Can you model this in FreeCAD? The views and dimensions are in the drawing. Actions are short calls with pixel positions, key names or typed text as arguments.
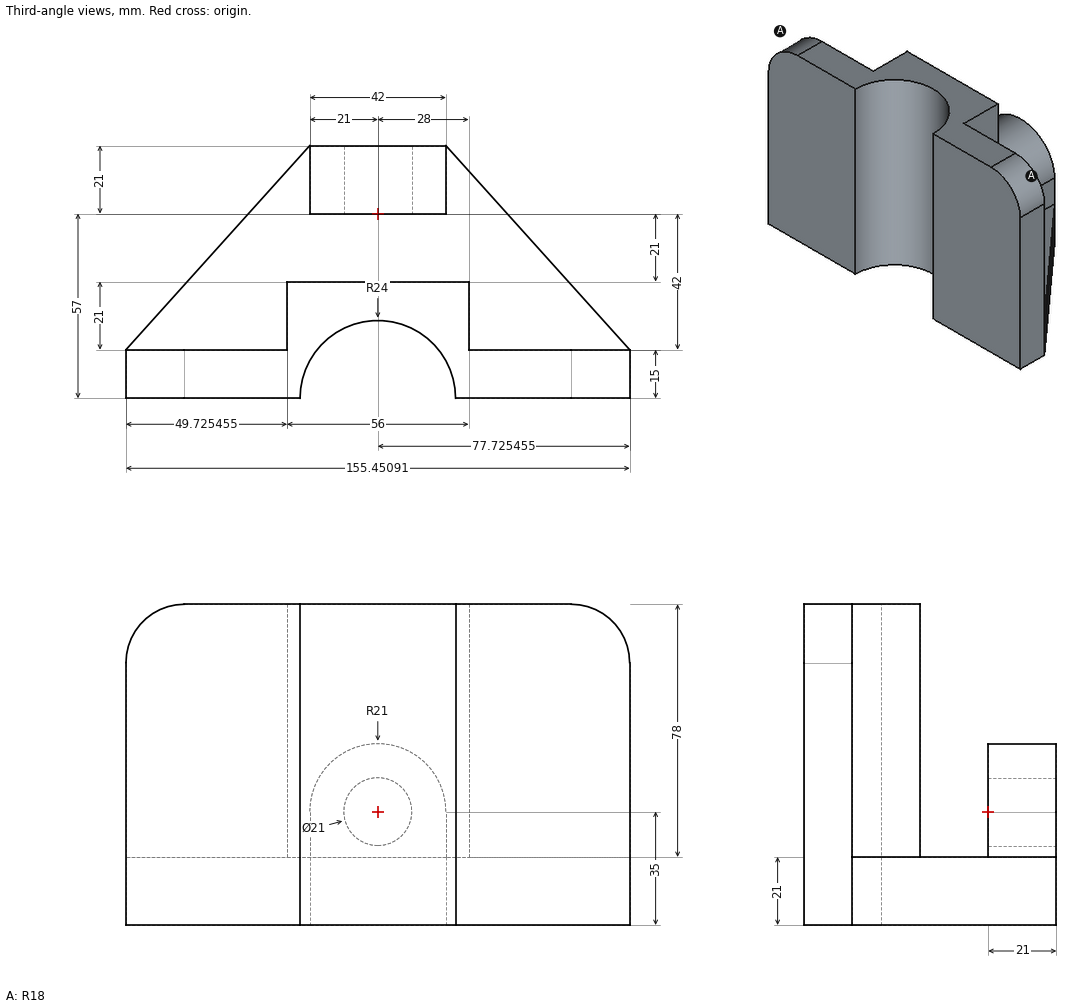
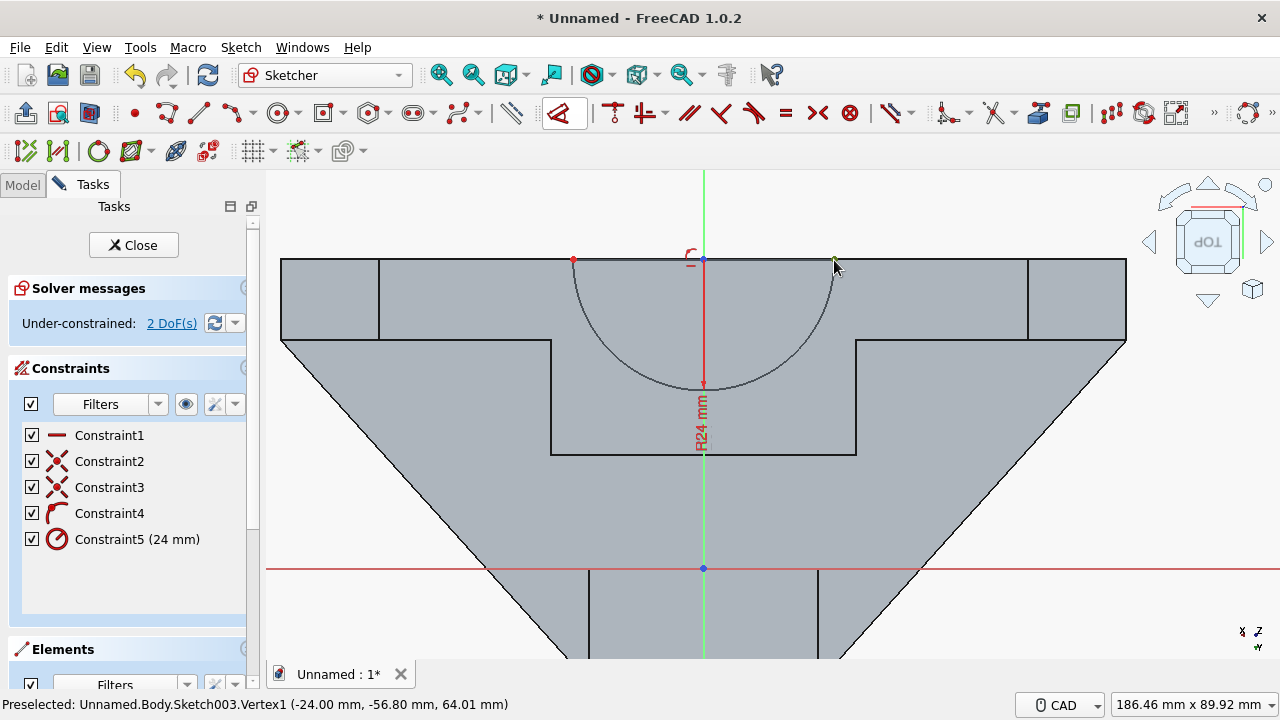
click(582, 114)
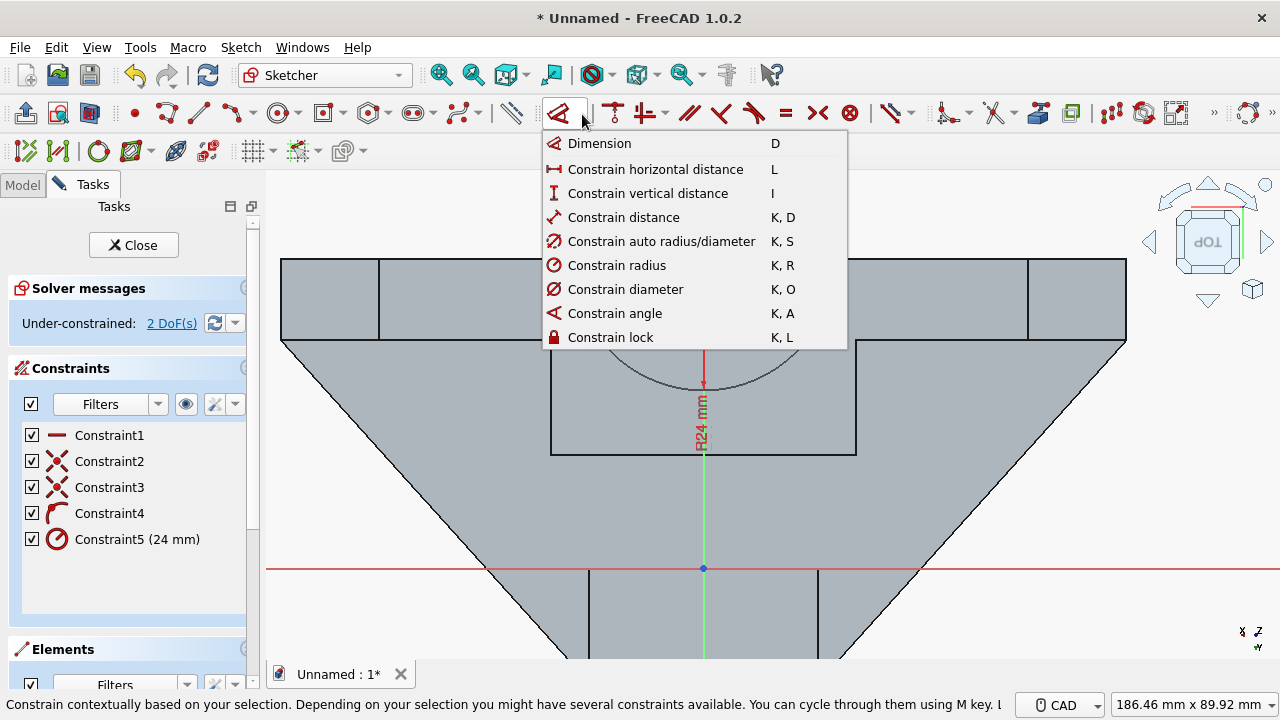
click(695, 193)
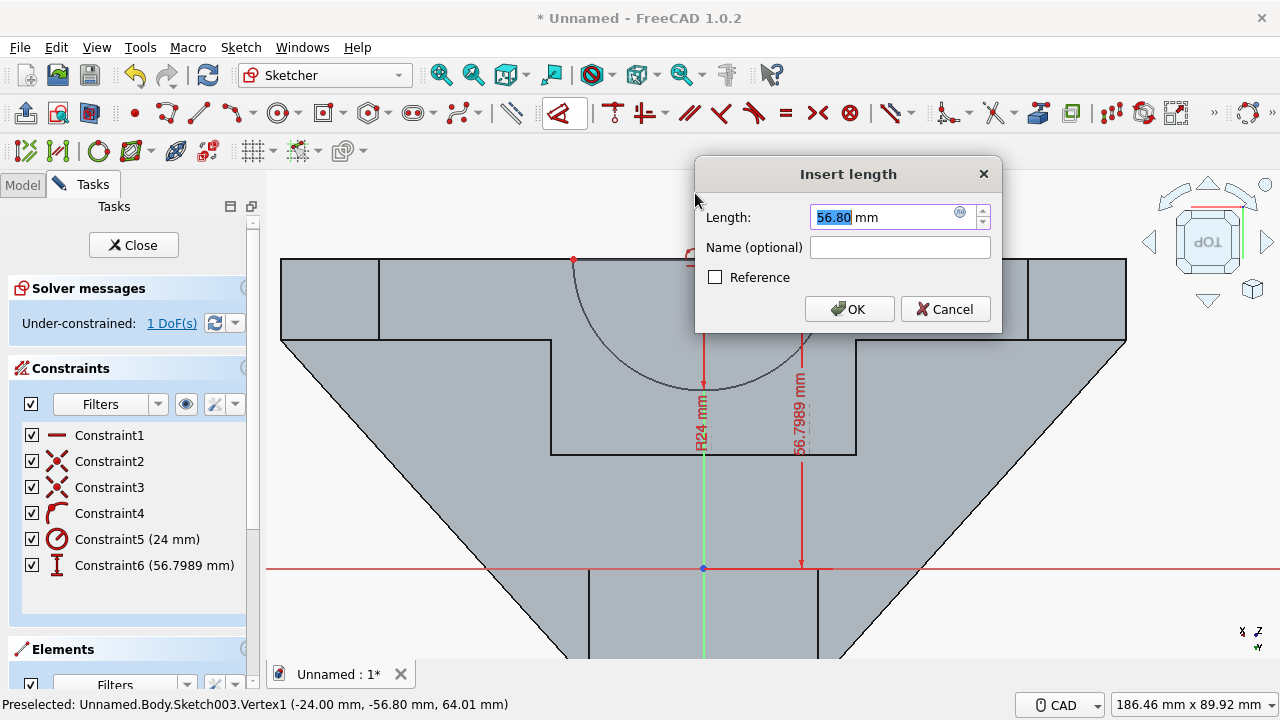
text(57)
key(Return)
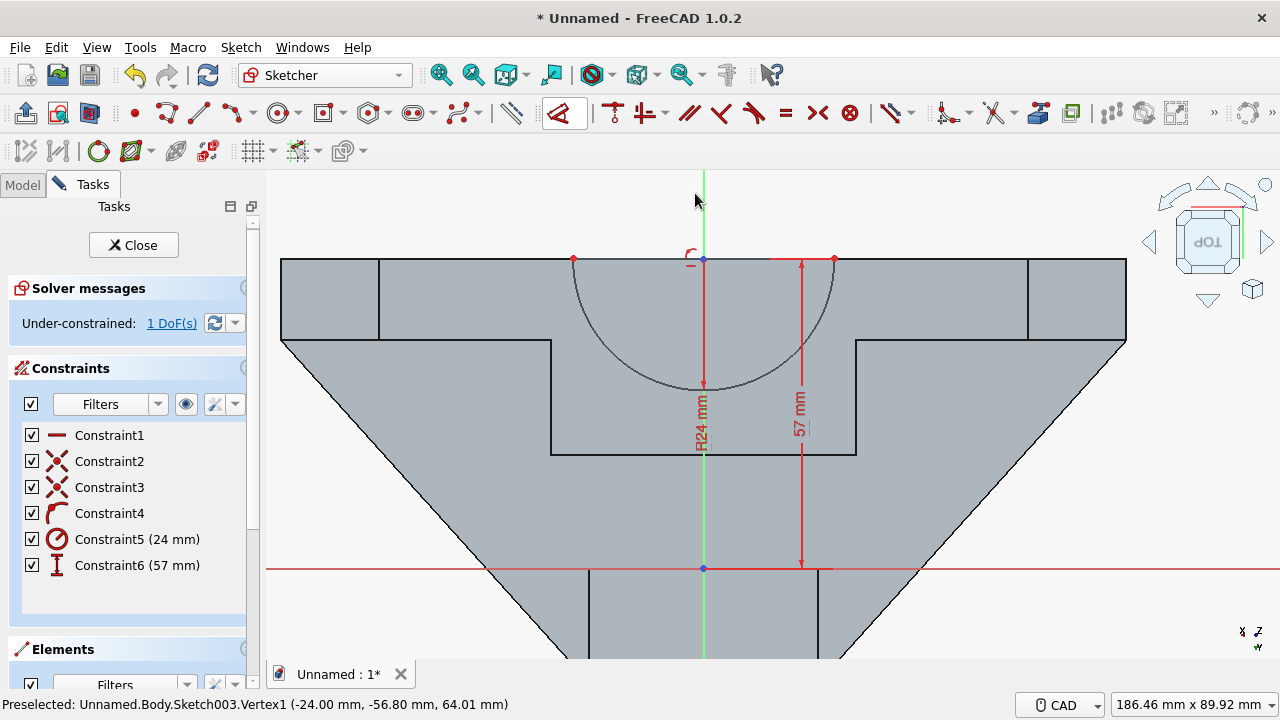
click(704, 260)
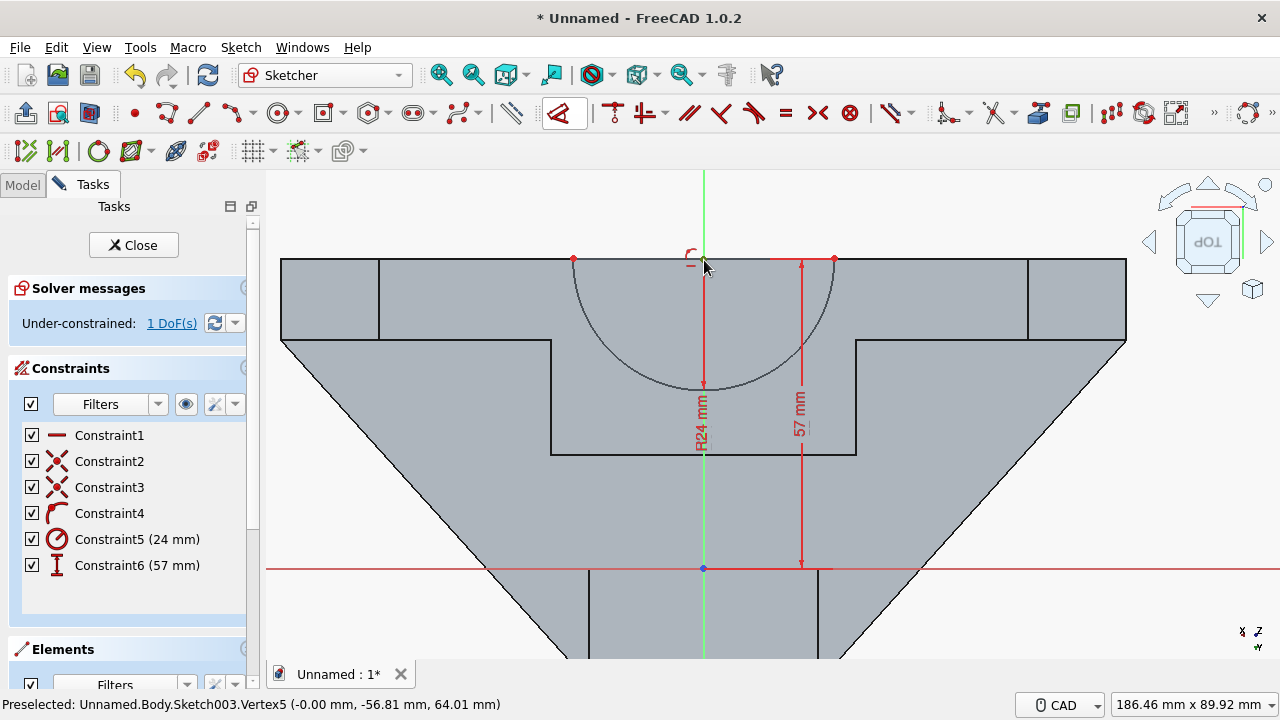
click(582, 114)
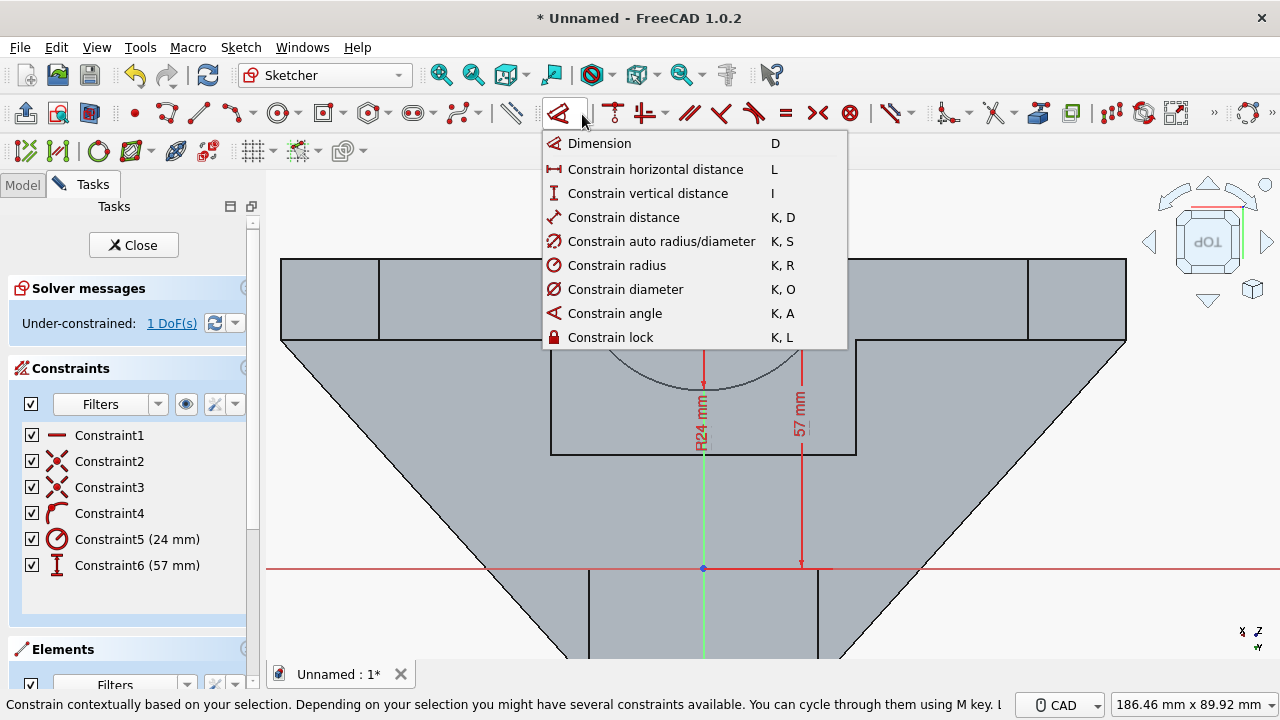
click(695, 193)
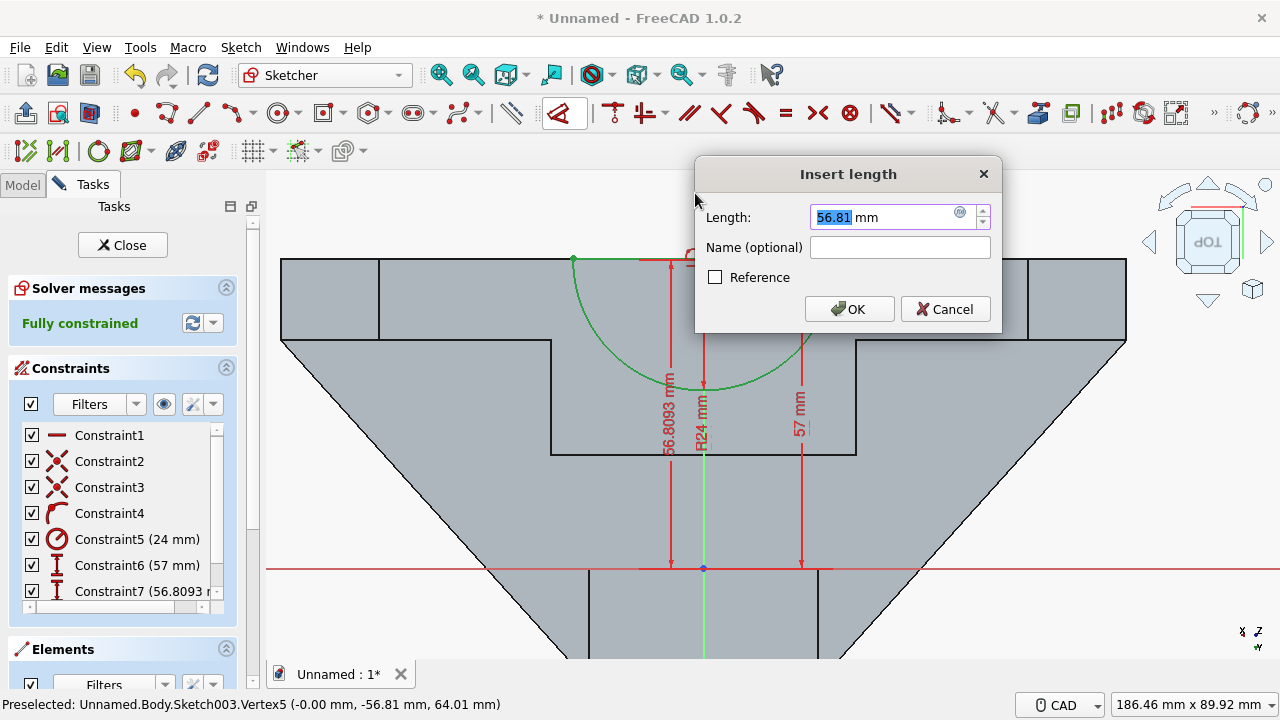
text(57)
key(Return)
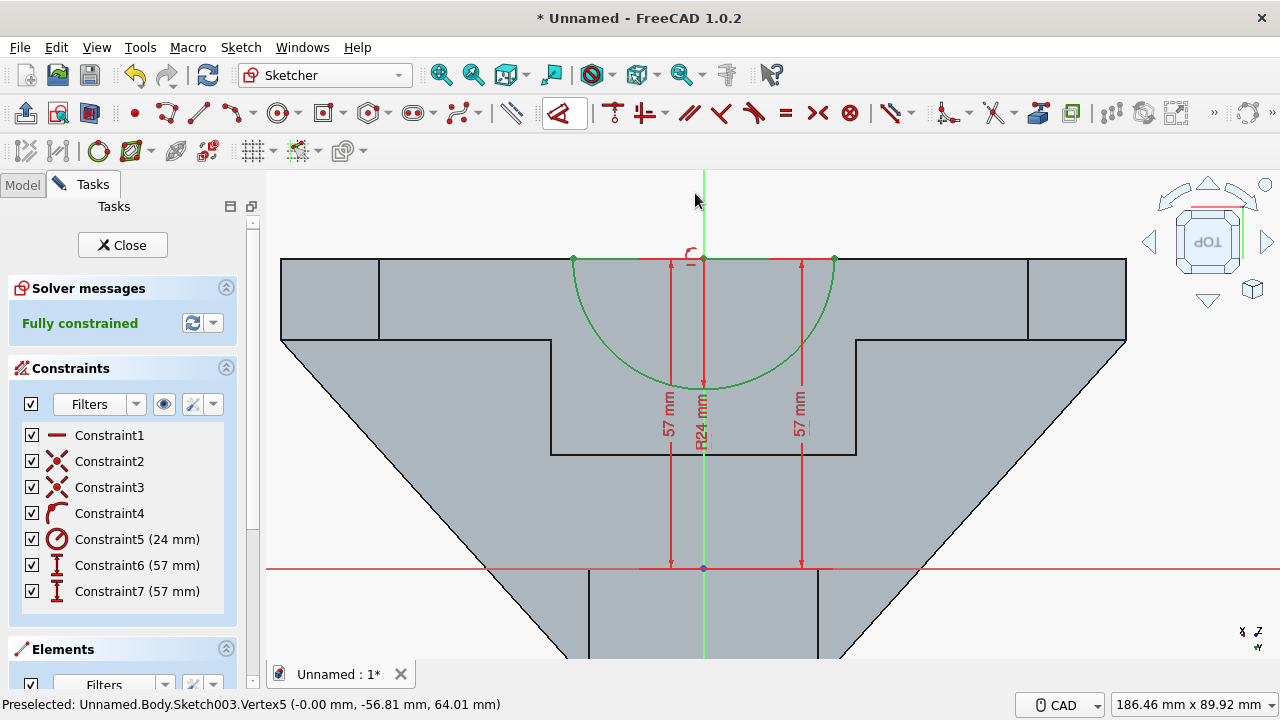
click(123, 245)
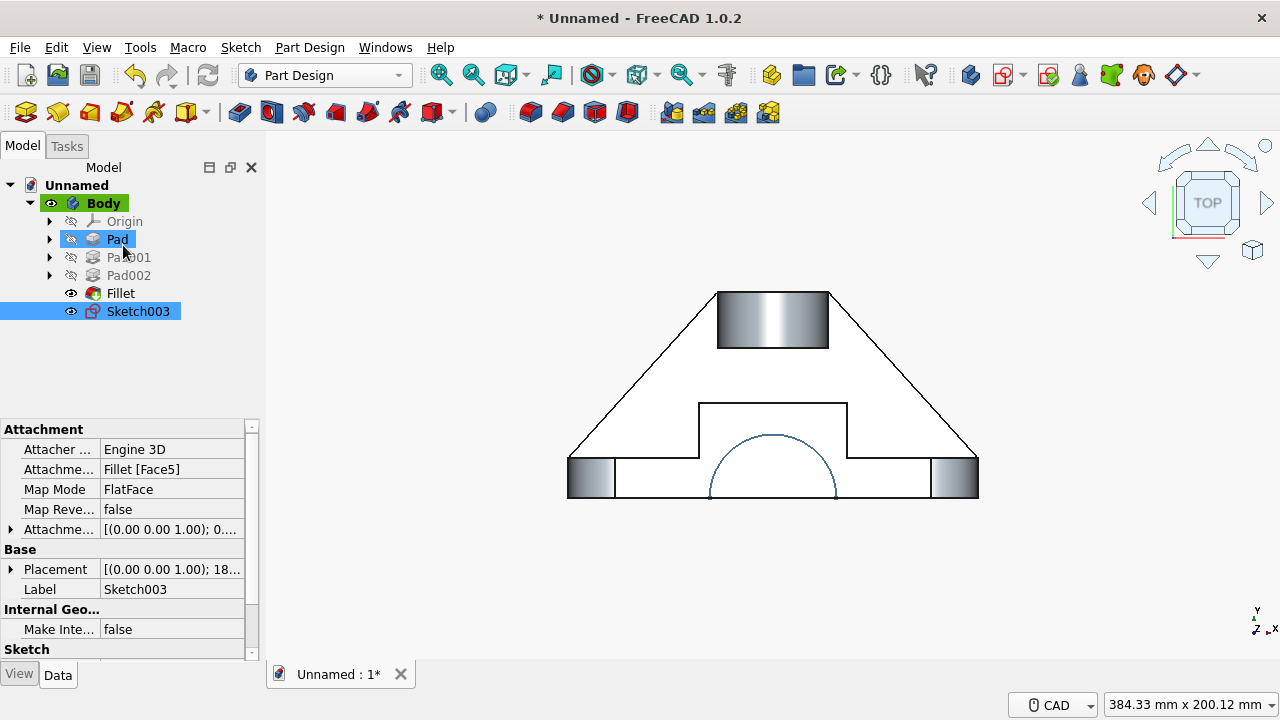
click(240, 112)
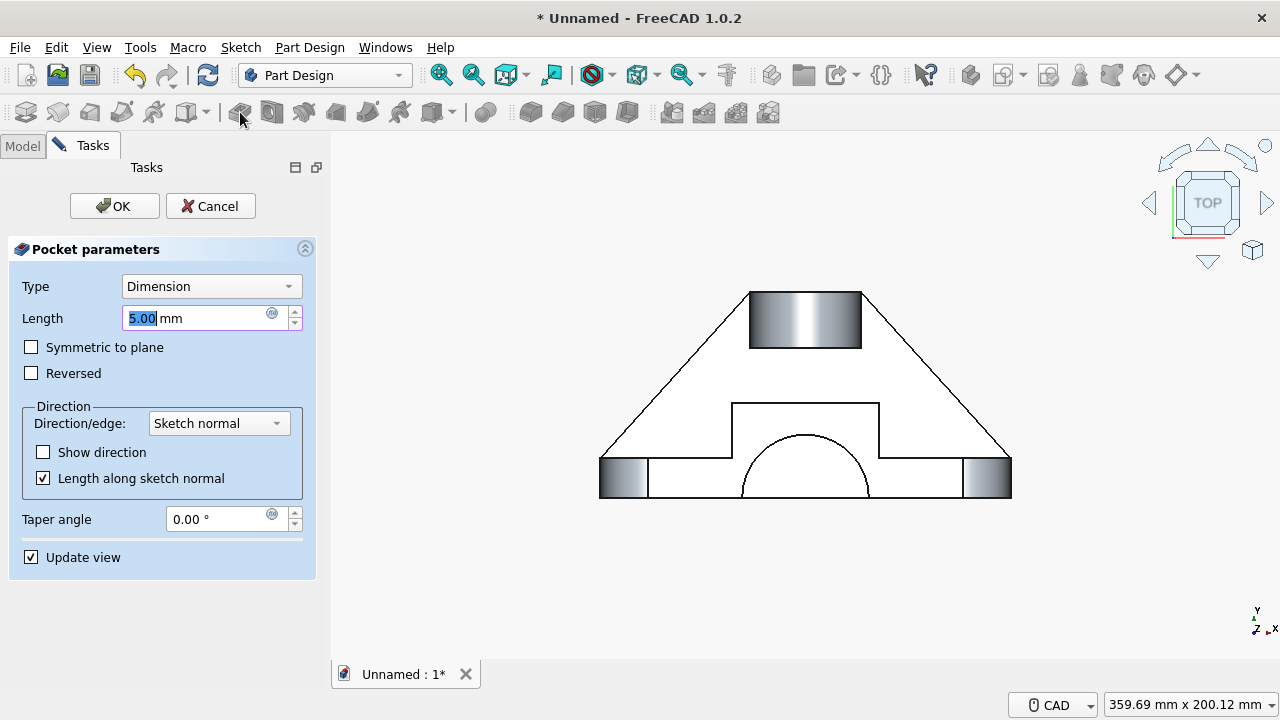
click(212, 286)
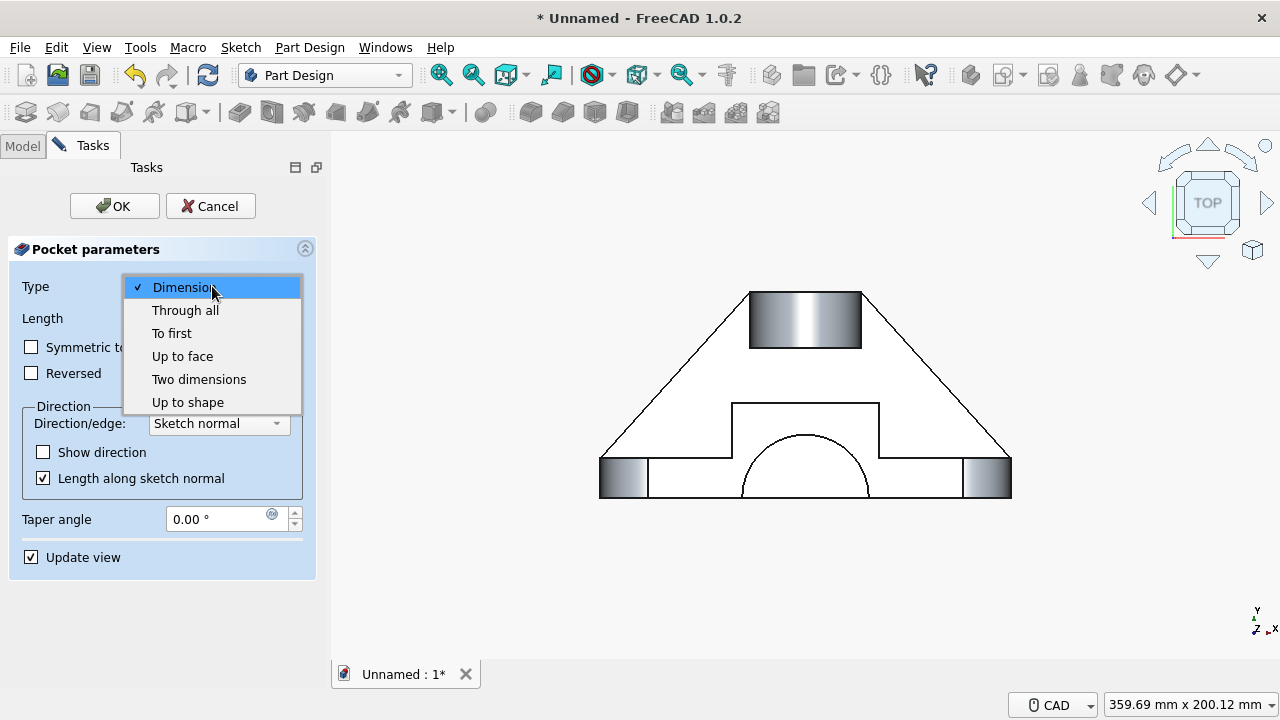
click(212, 334)